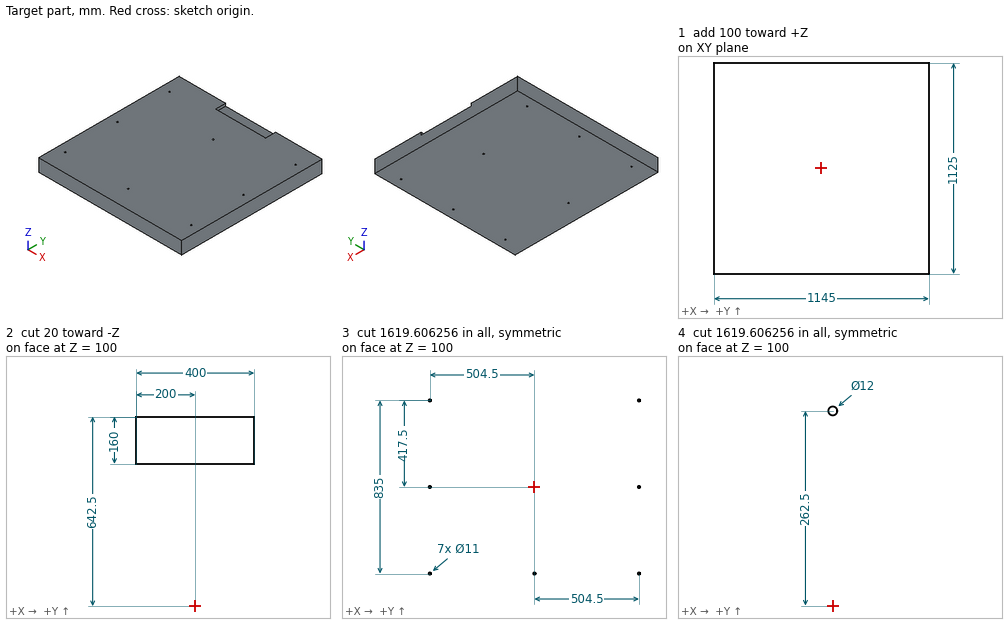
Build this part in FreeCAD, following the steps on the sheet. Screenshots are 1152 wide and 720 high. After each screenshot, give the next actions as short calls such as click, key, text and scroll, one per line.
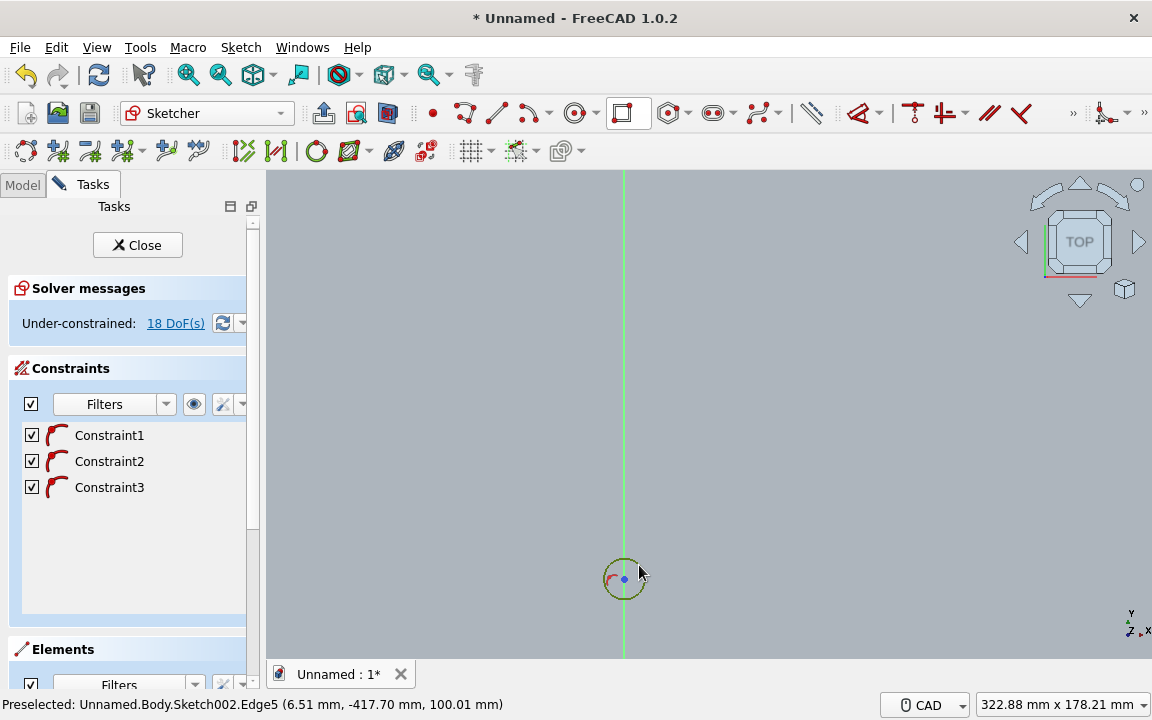
scroll(643, 570, down, 10)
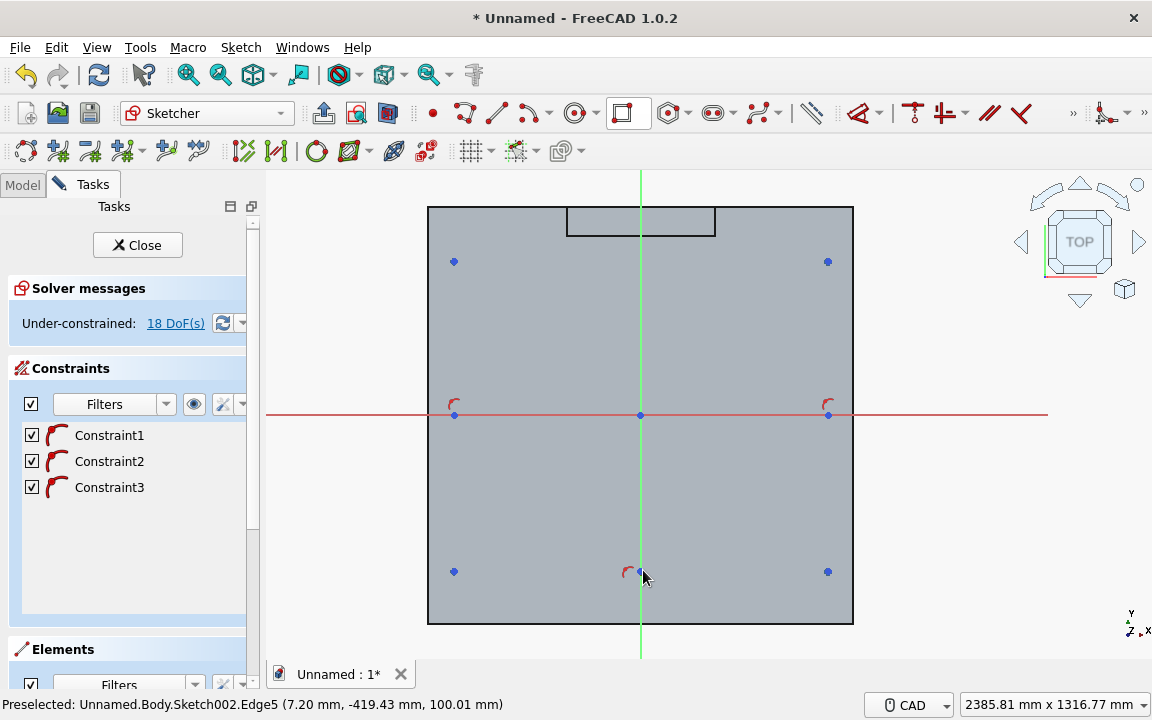
scroll(455, 414, up, 12)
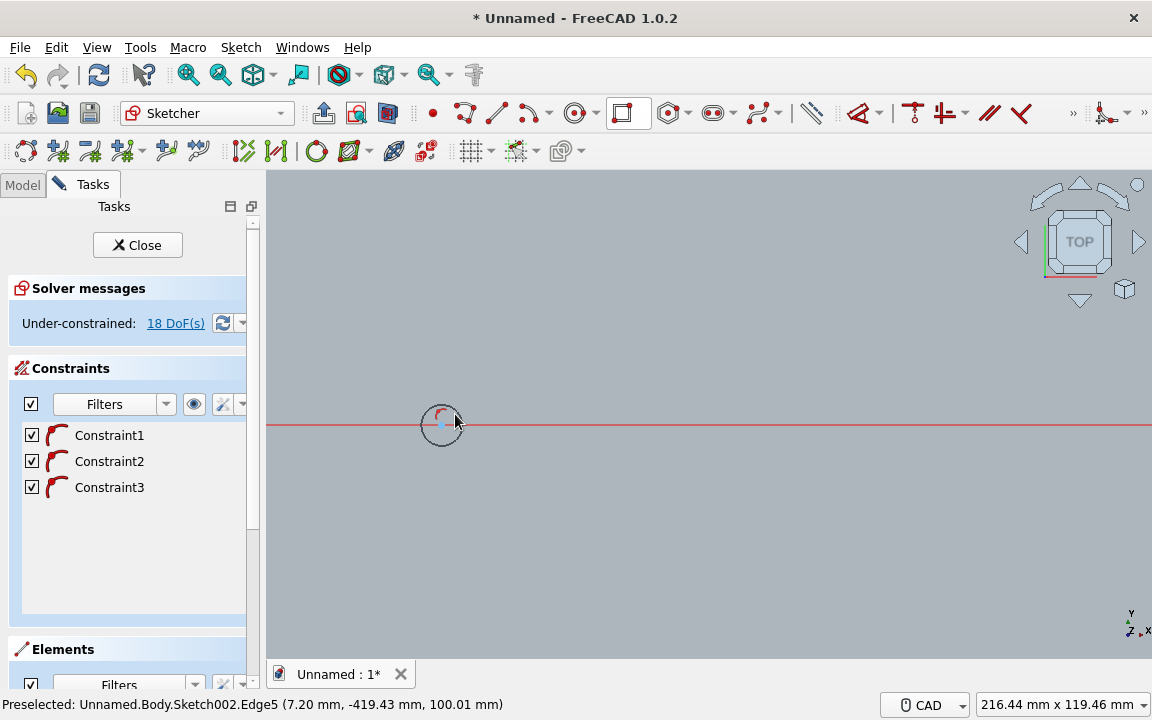
click(456, 411)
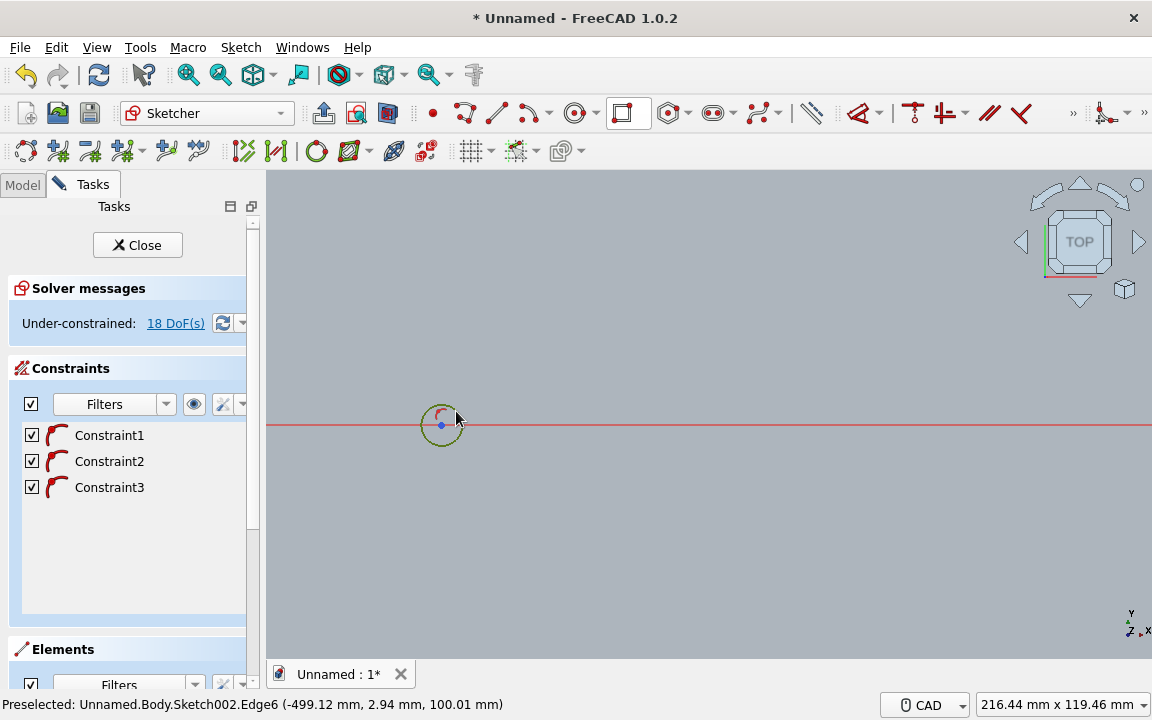
scroll(455, 413, down, 12)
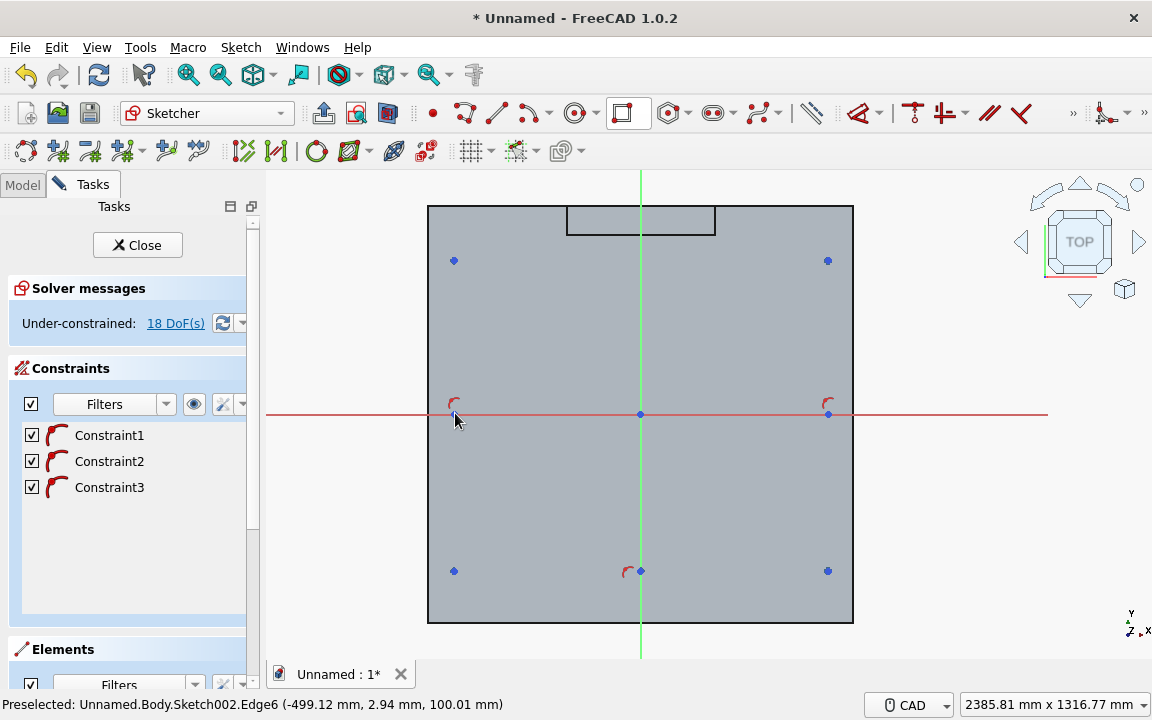
scroll(829, 413, up, 12)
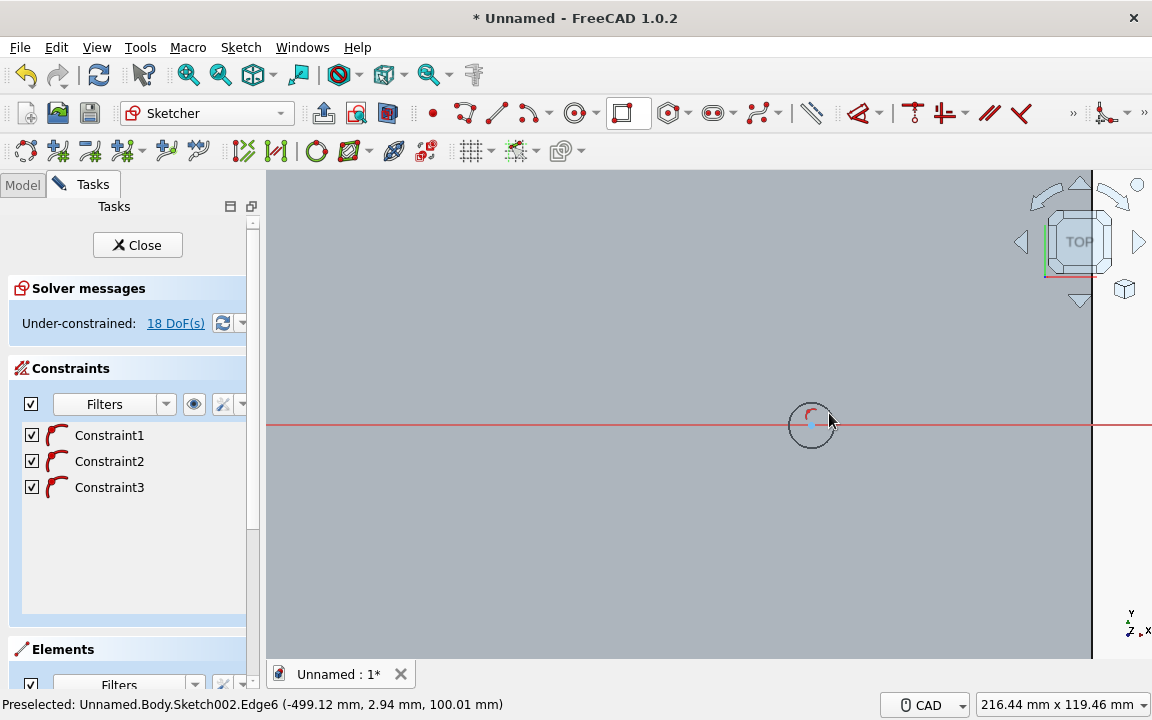
click(828, 409)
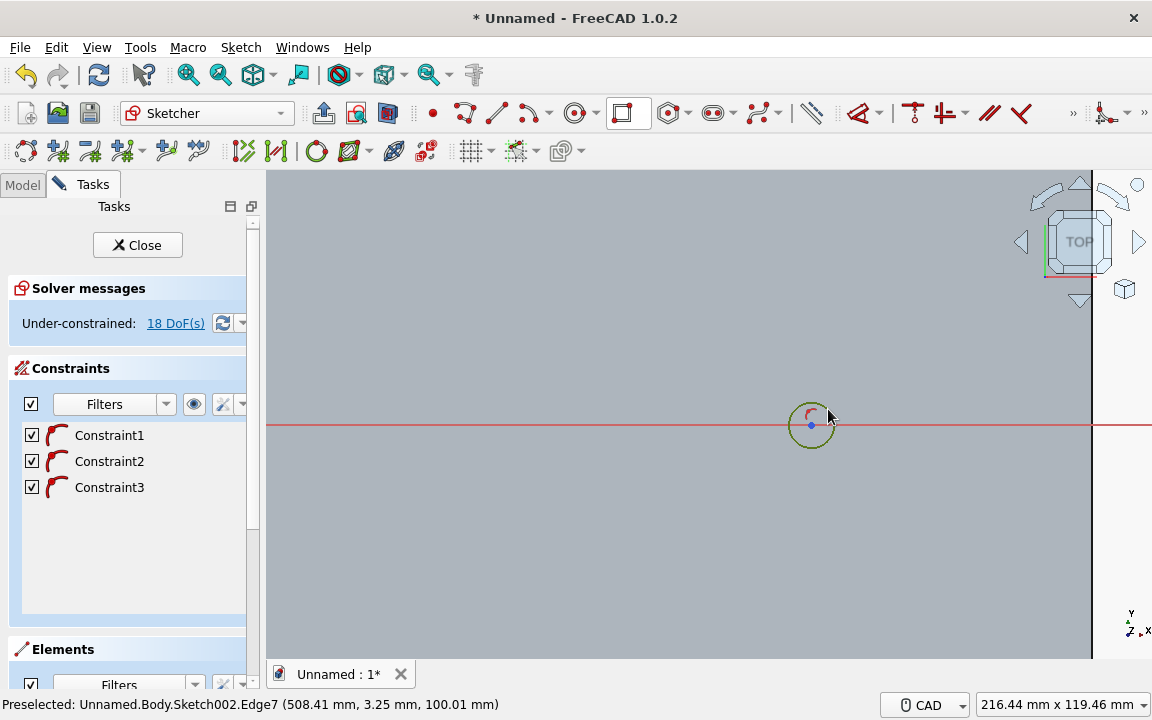
key(e)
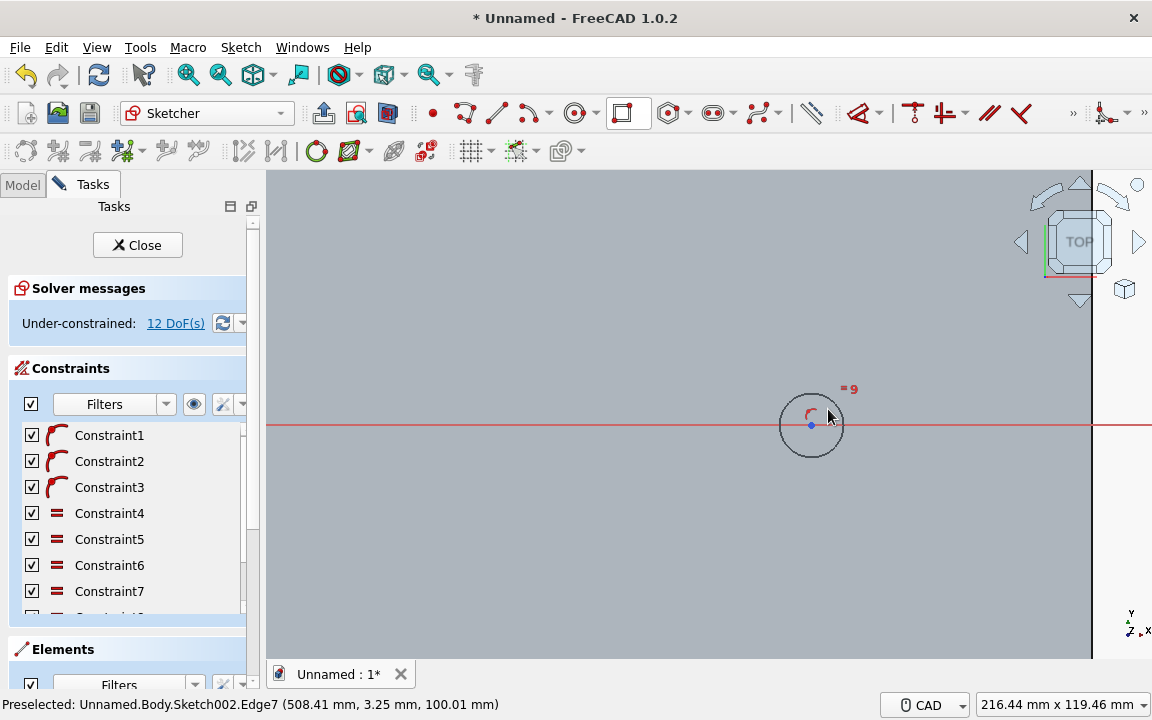
scroll(829, 413, down, 12)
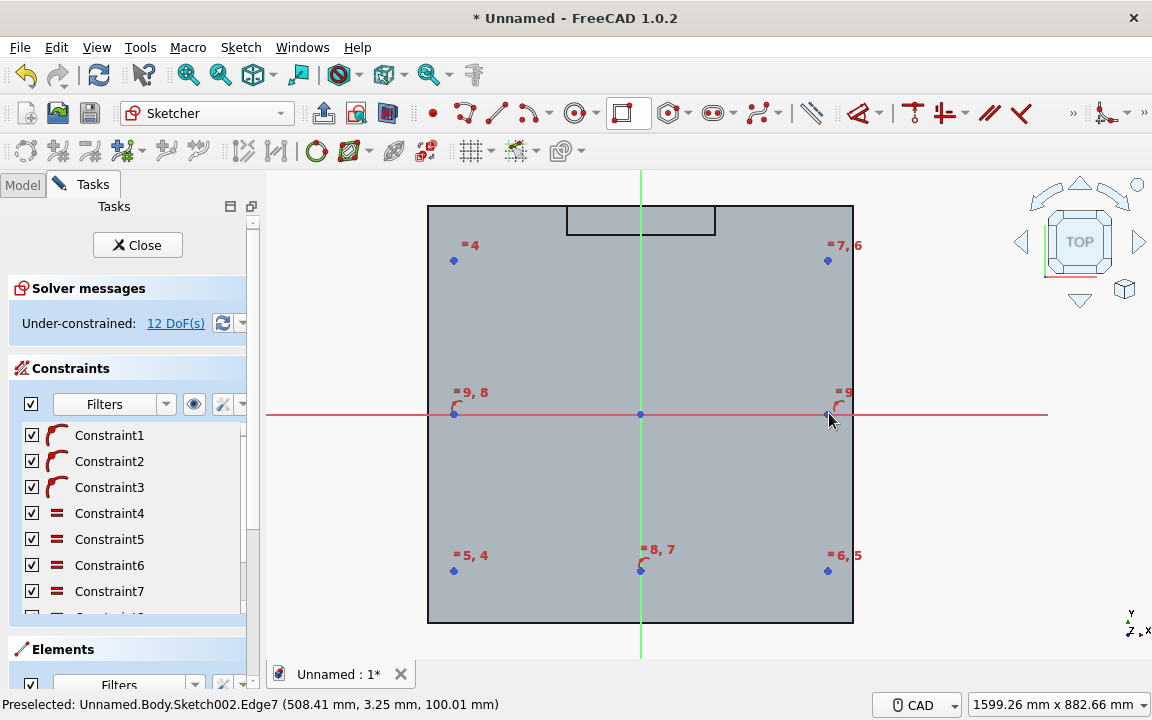
click(454, 261)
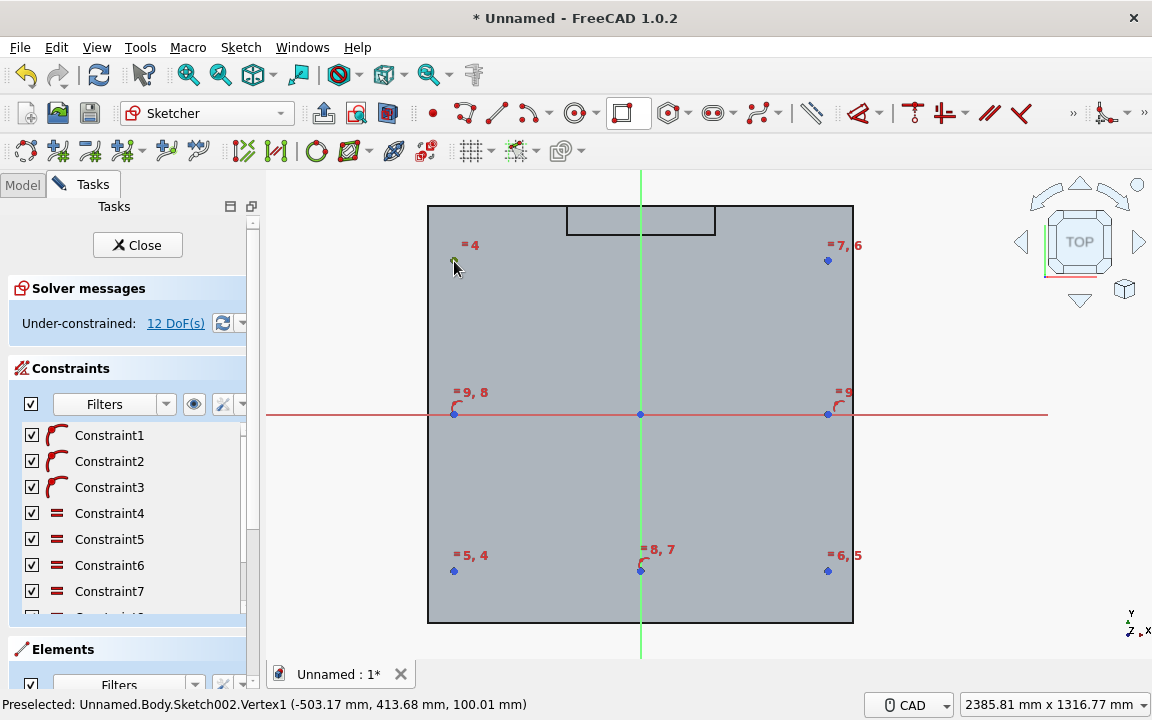
click(454, 571)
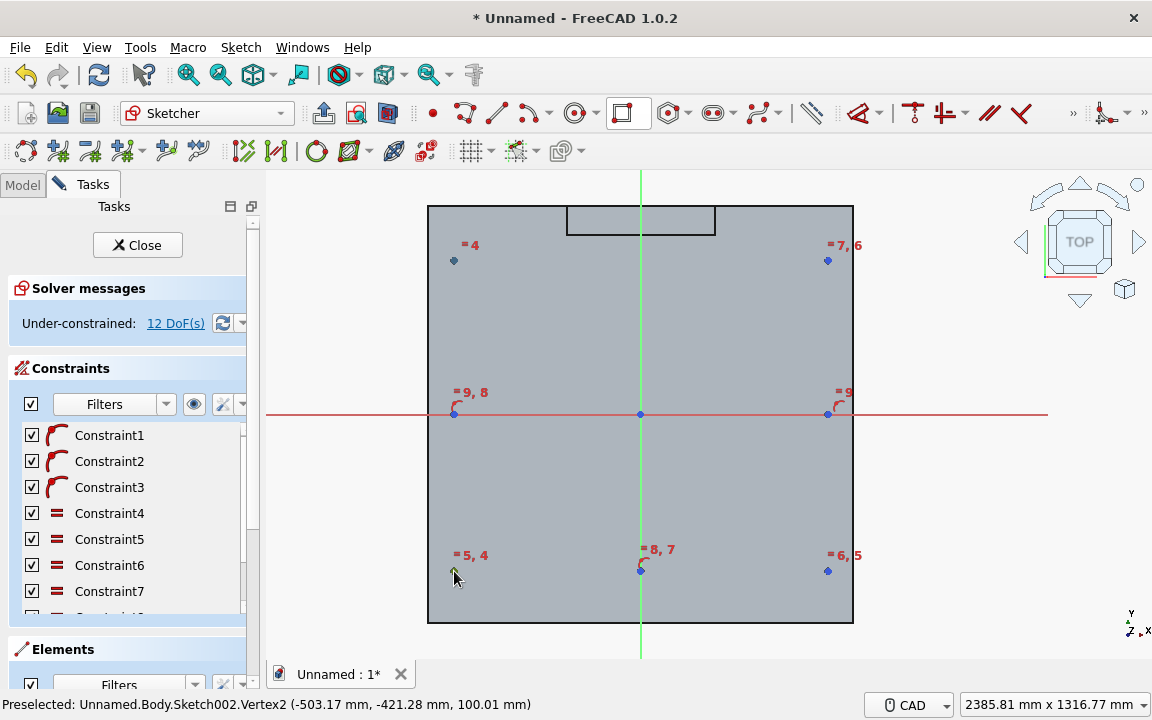
click(968, 114)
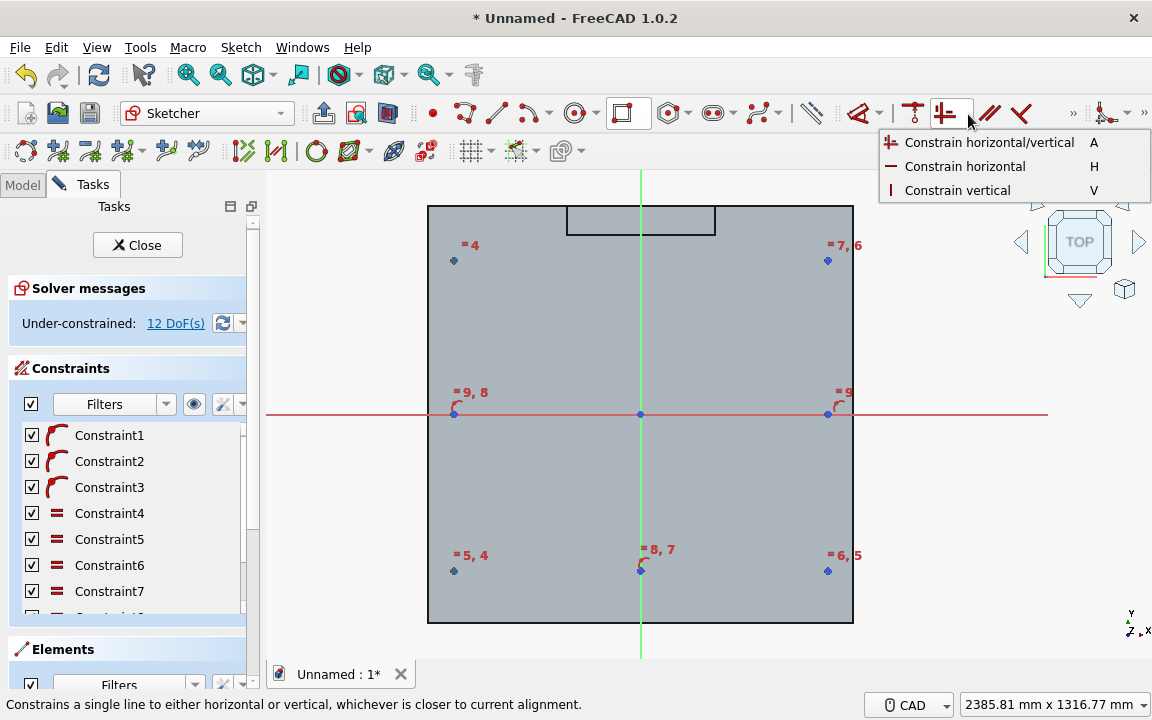
click(1015, 190)